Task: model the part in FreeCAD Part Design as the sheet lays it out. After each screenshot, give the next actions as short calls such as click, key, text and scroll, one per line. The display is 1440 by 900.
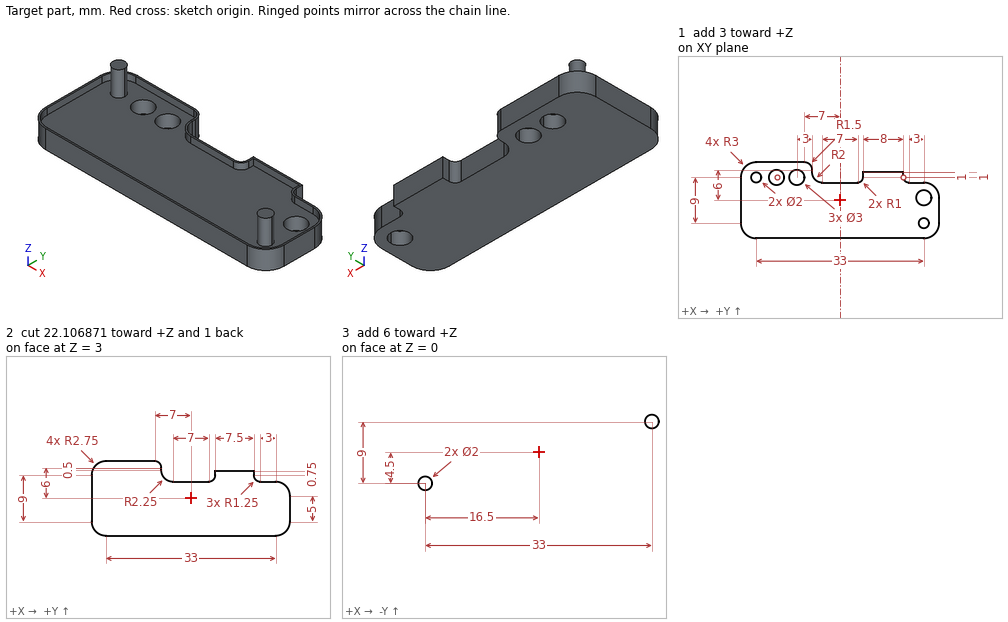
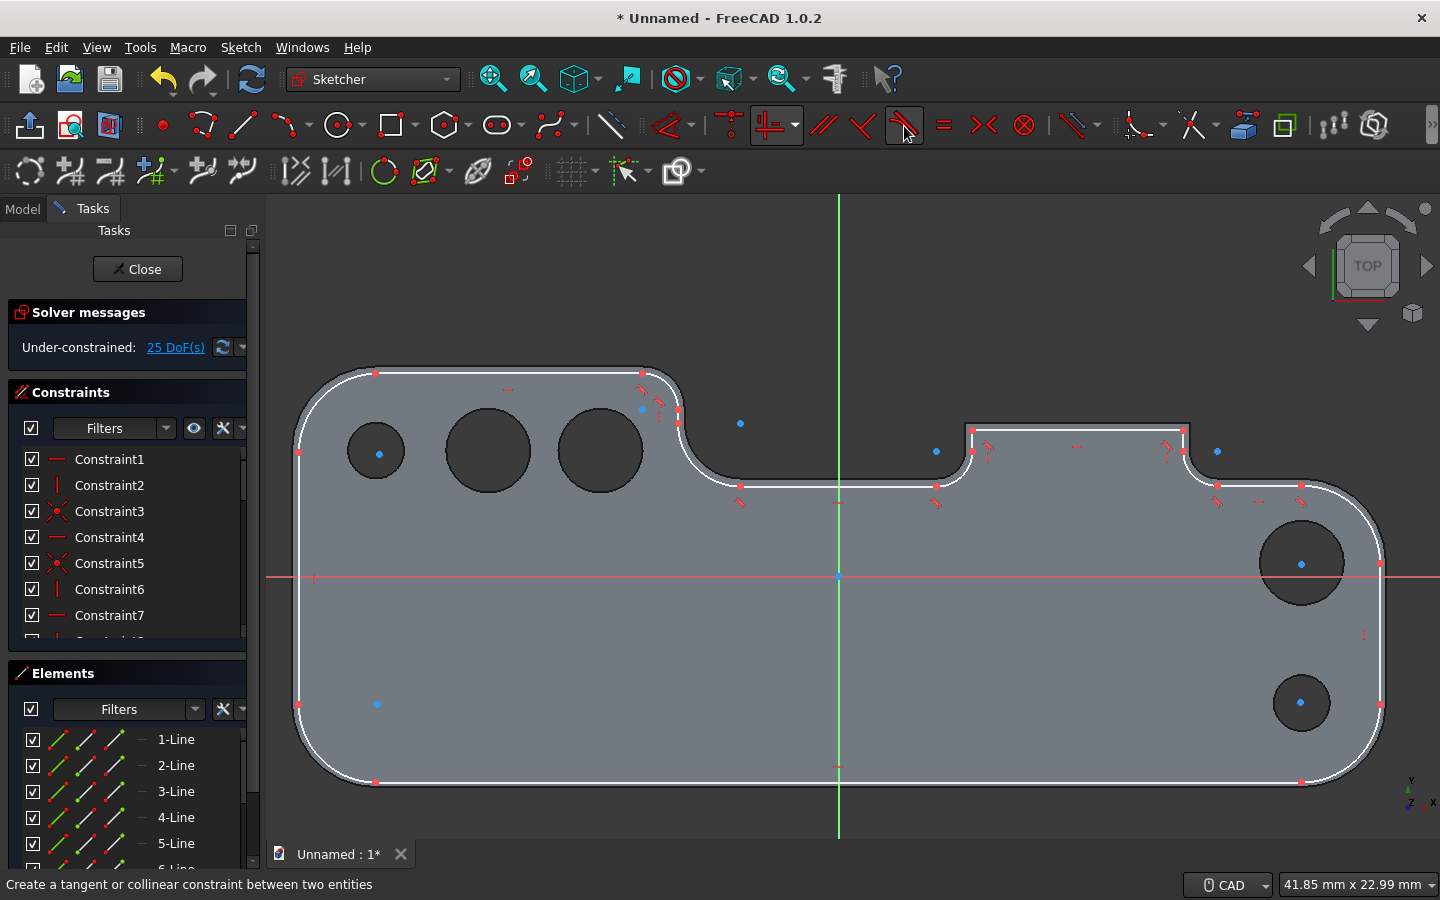
click(562, 373)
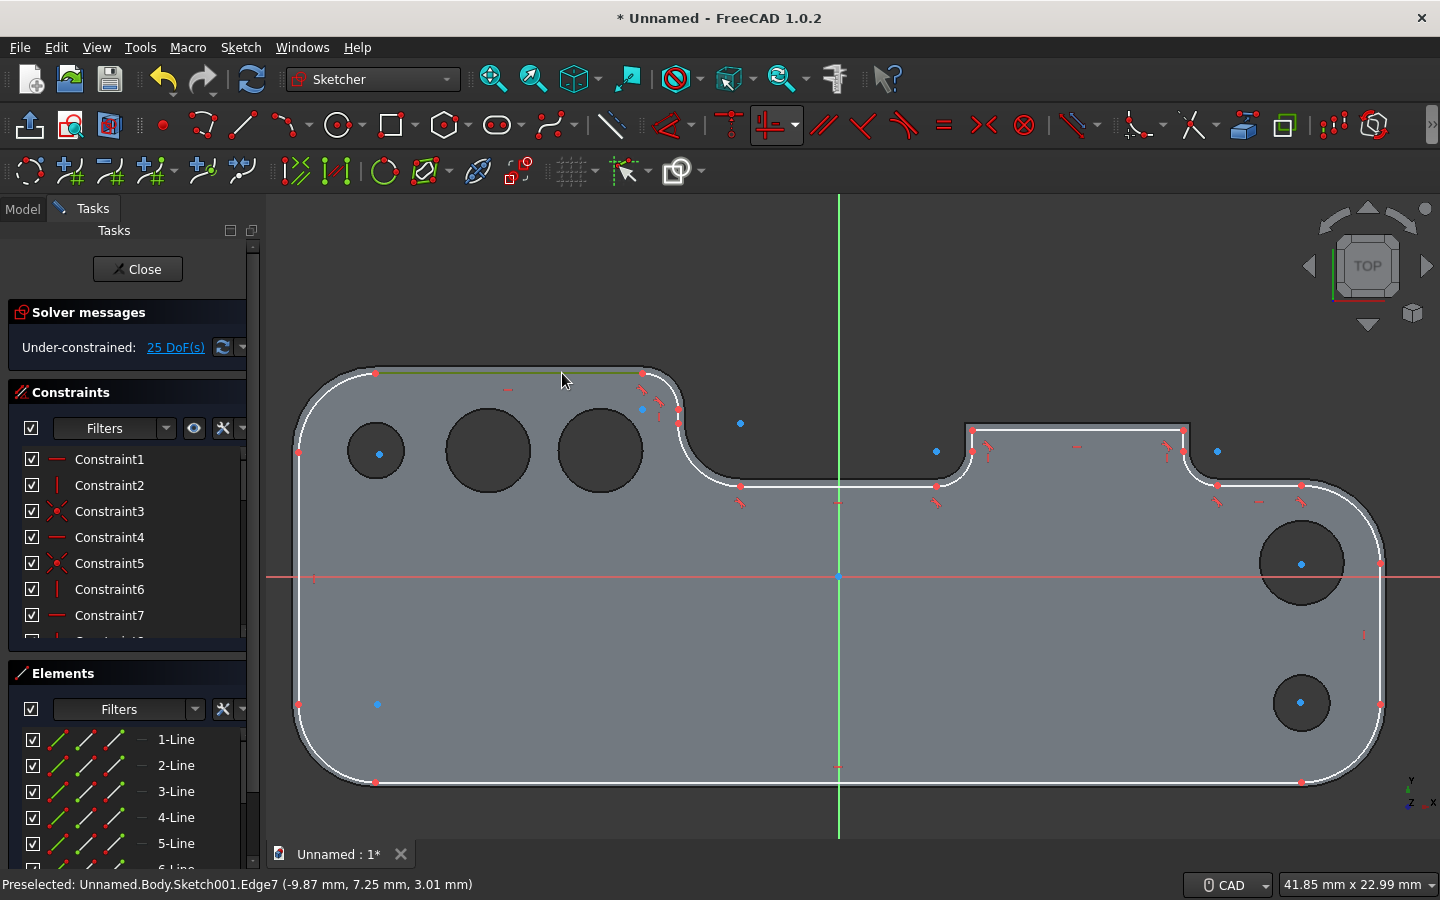
click(341, 383)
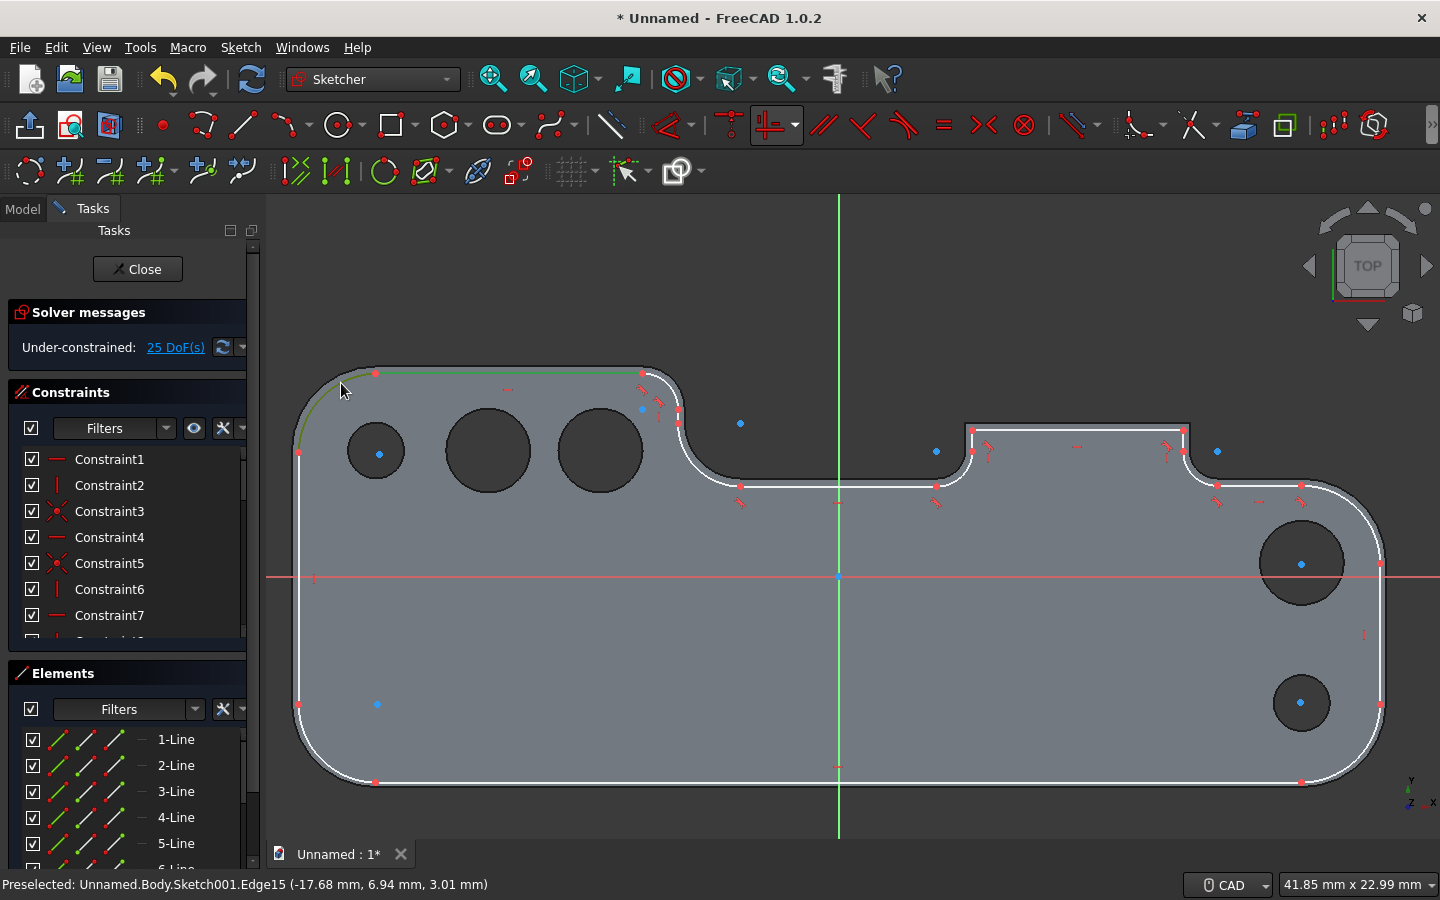
click(904, 126)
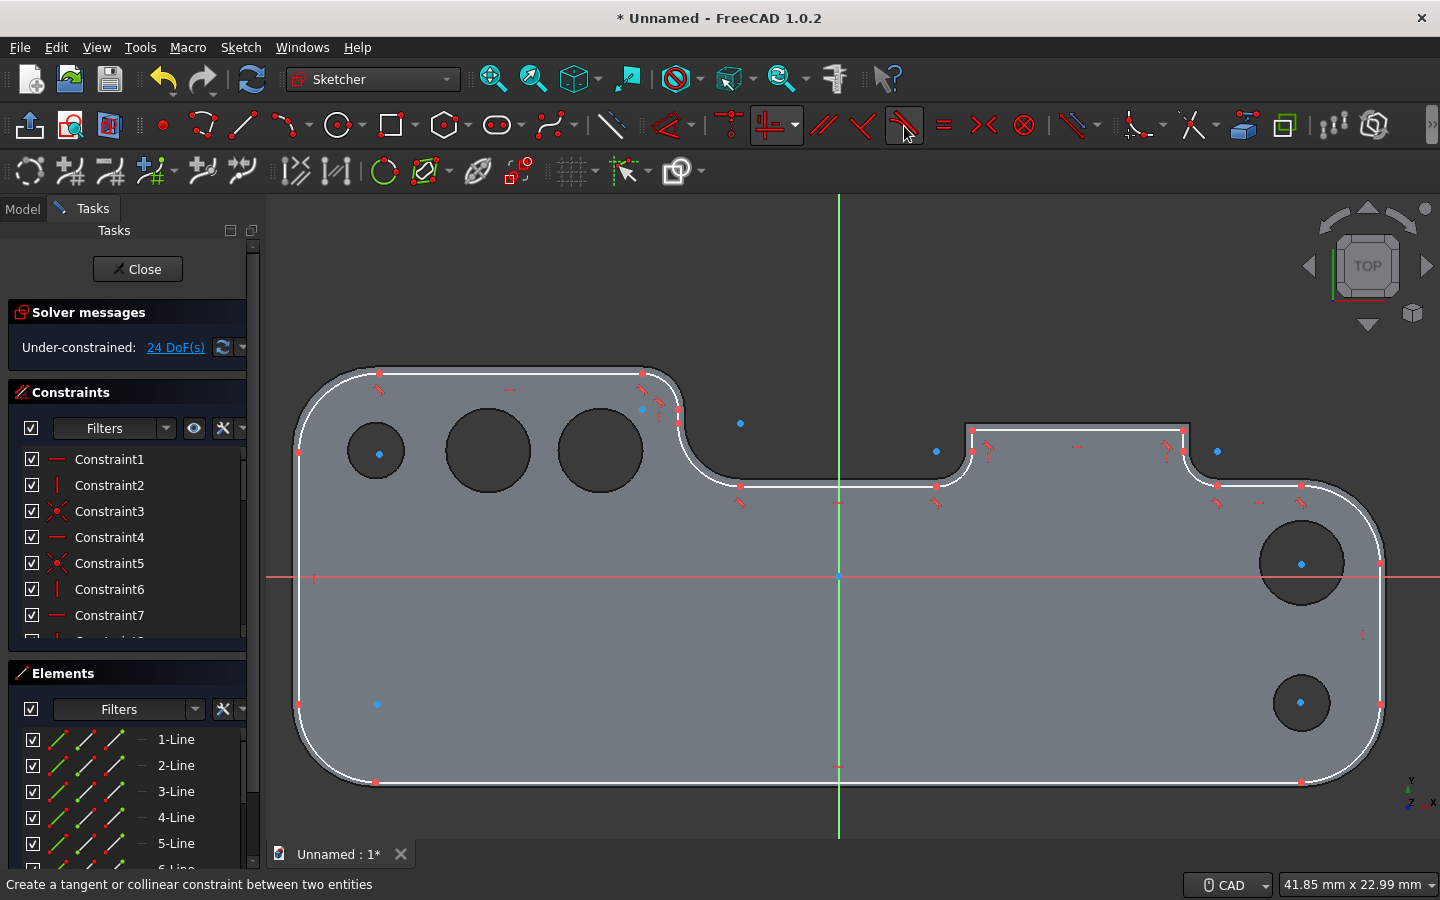
click(299, 528)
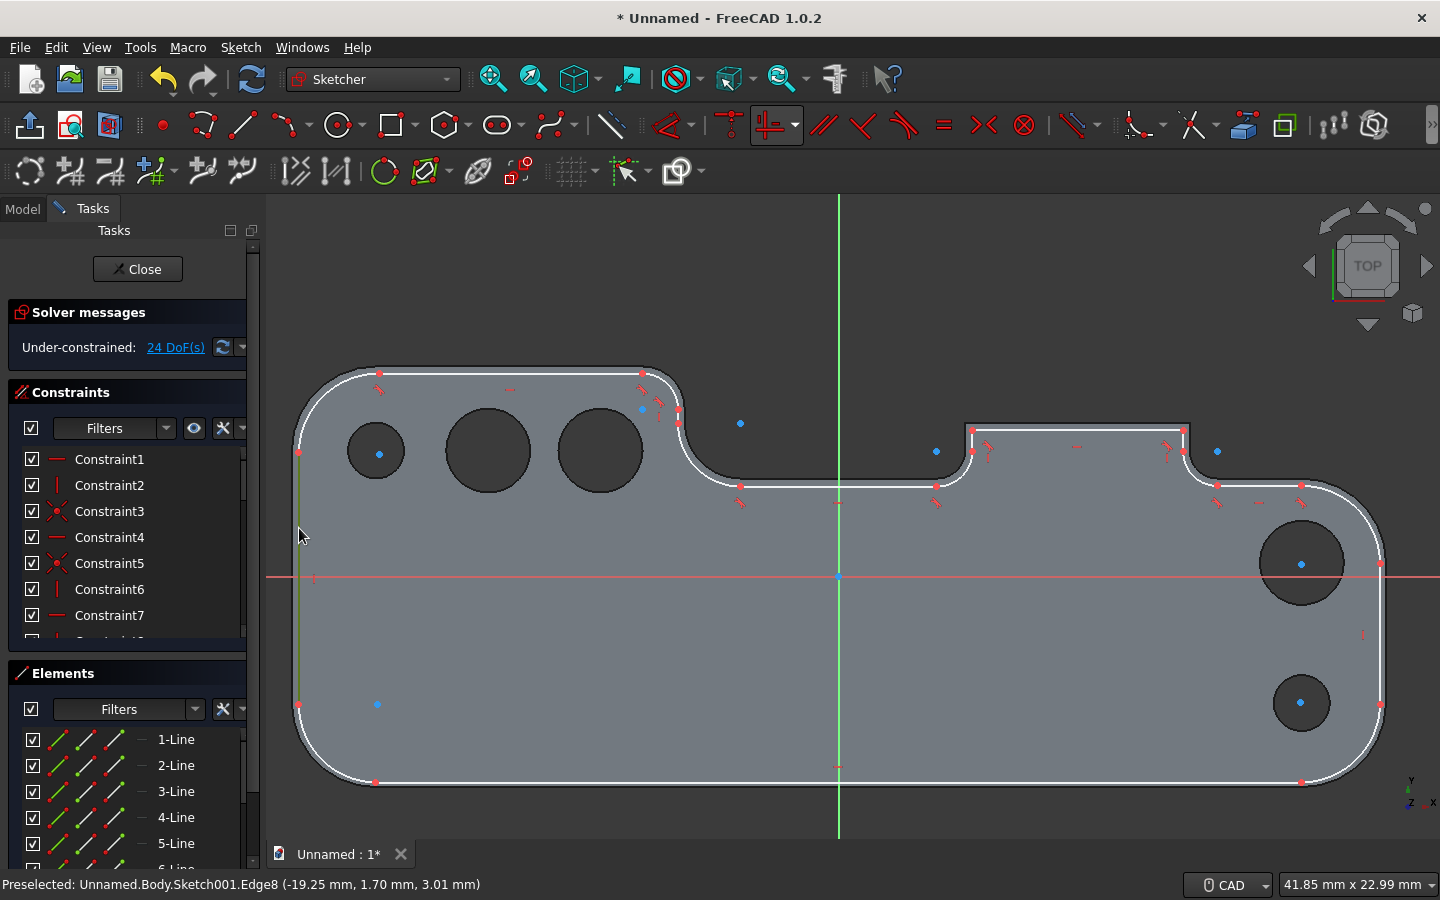
click(343, 382)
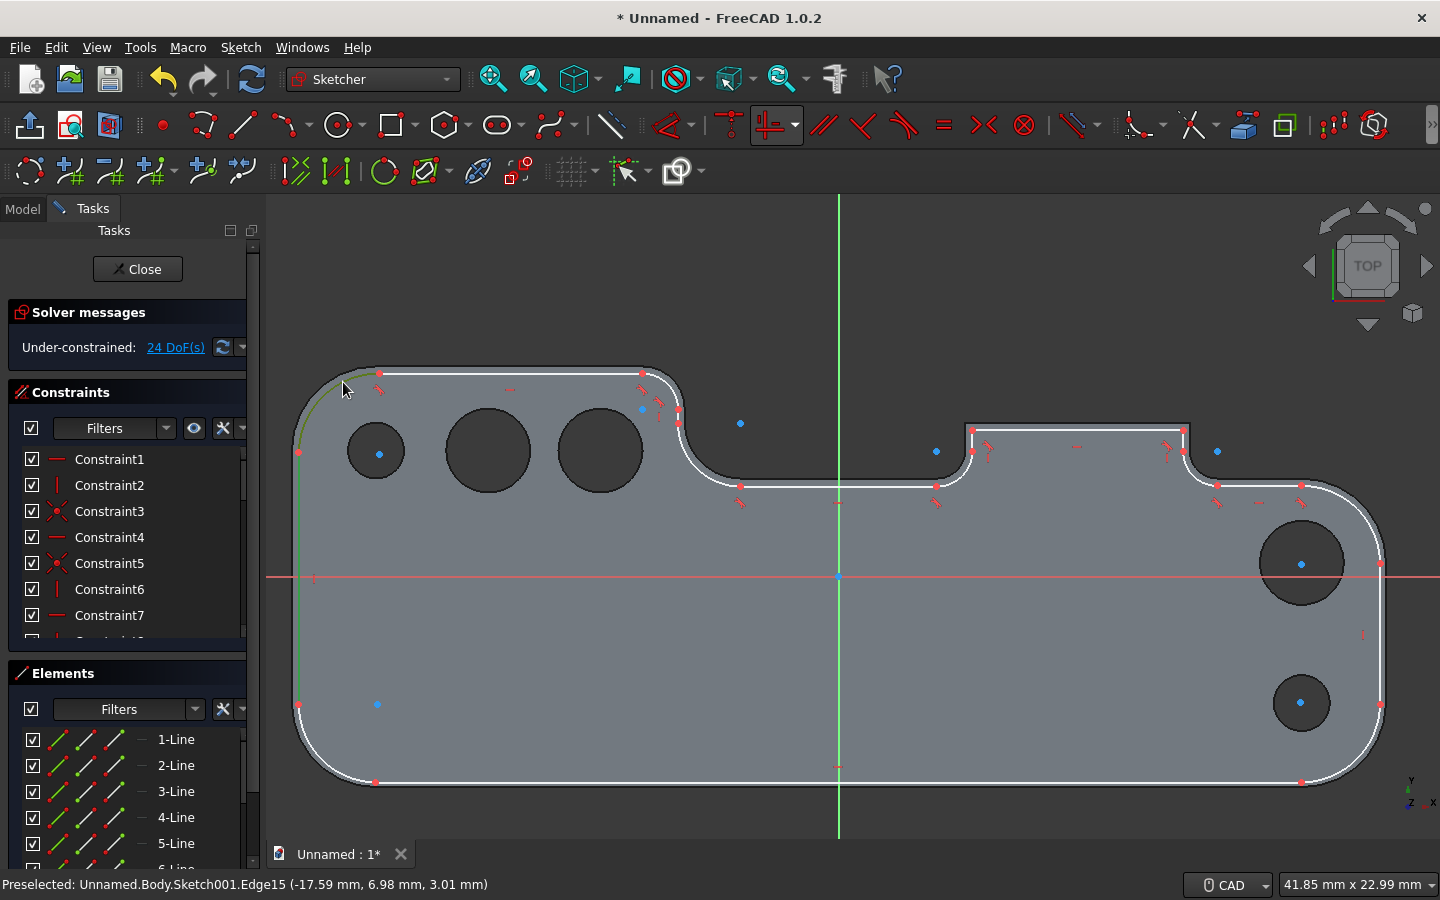
click(904, 126)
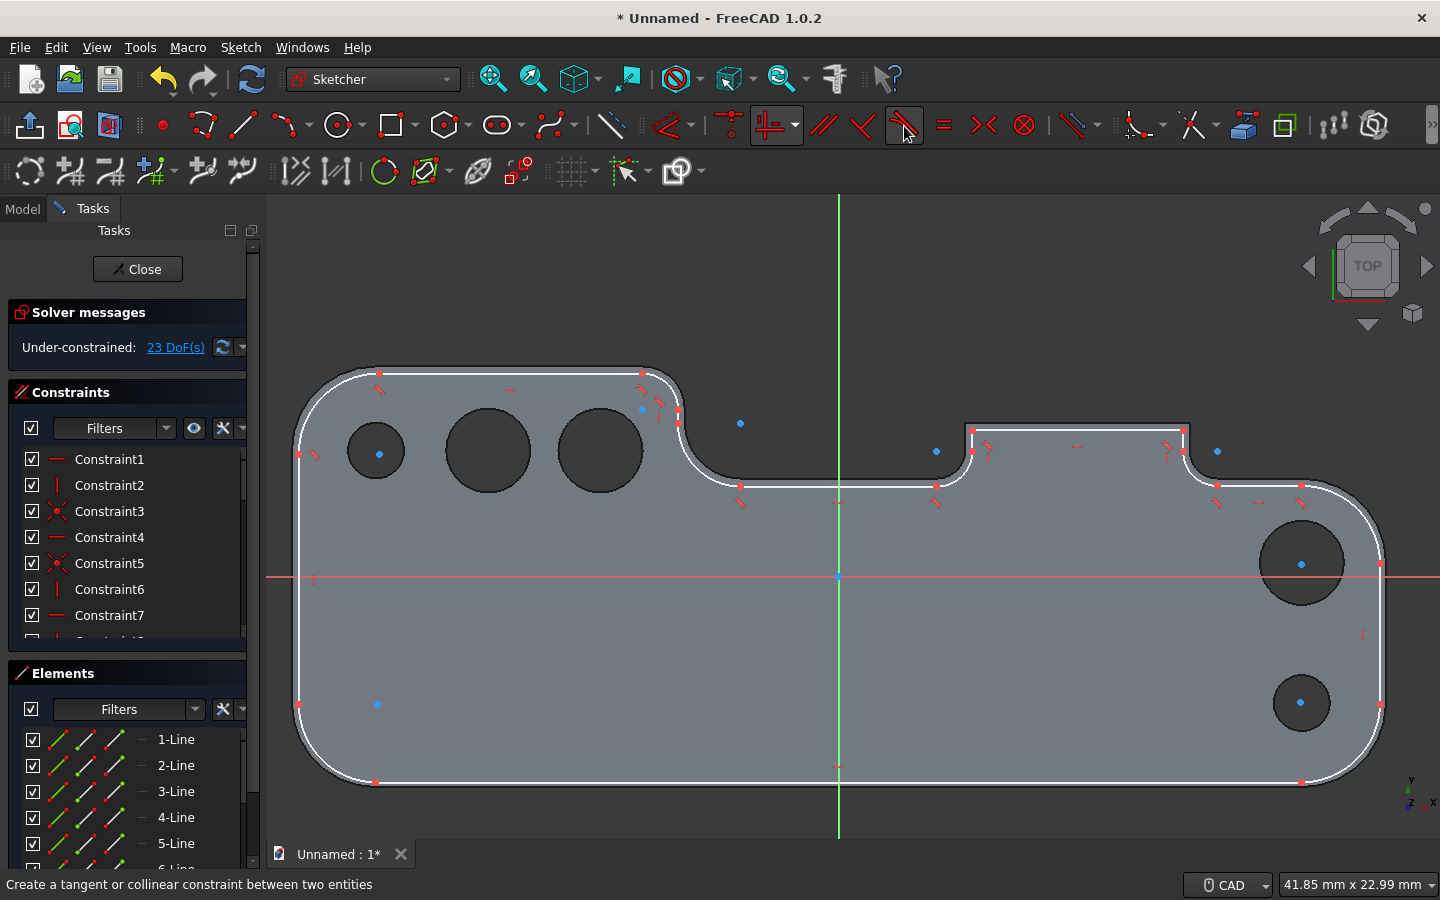
click(299, 529)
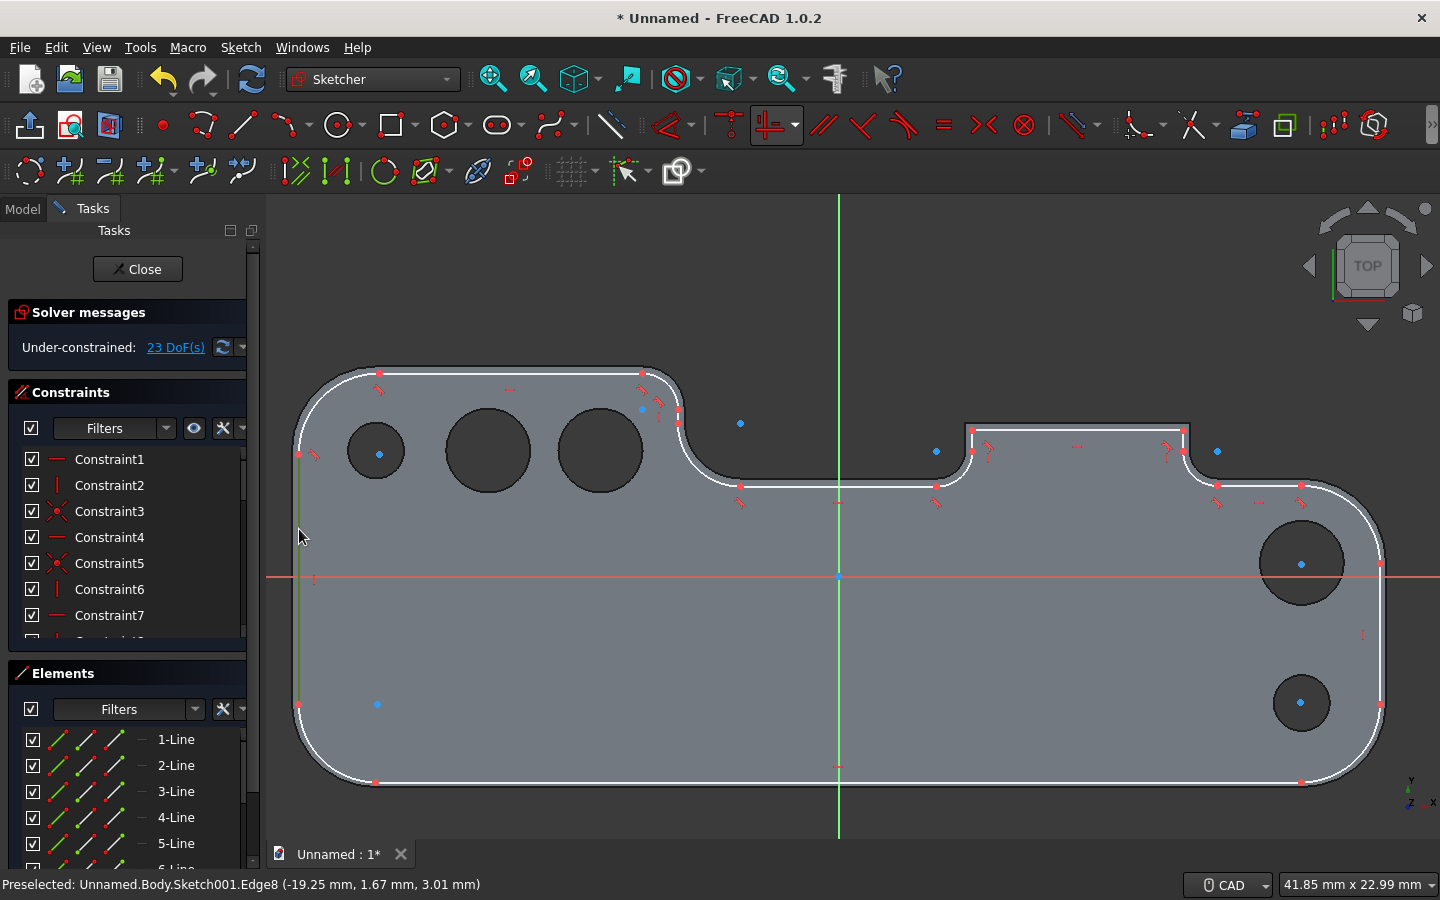
click(307, 739)